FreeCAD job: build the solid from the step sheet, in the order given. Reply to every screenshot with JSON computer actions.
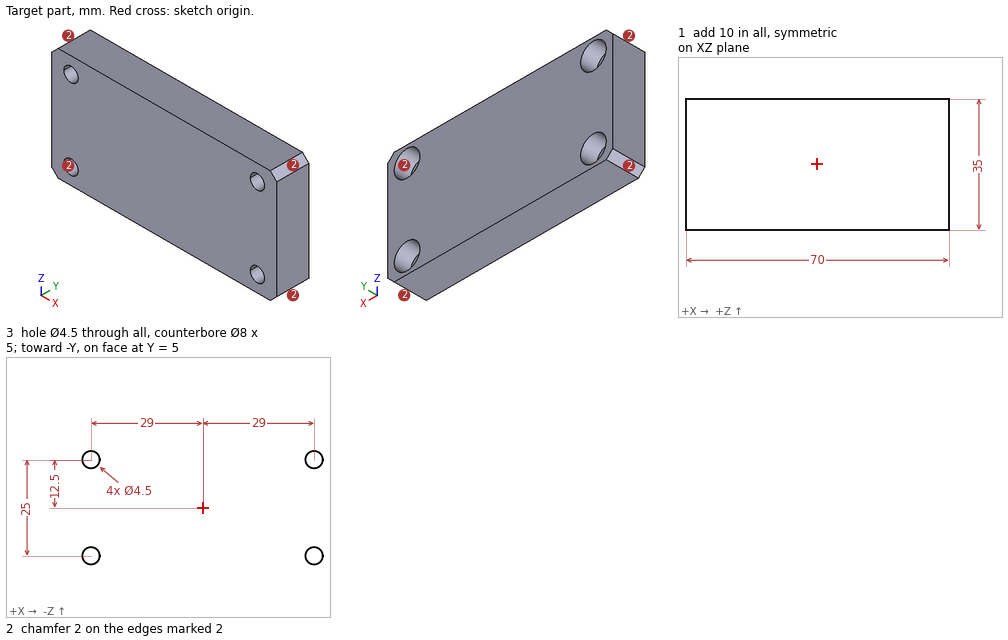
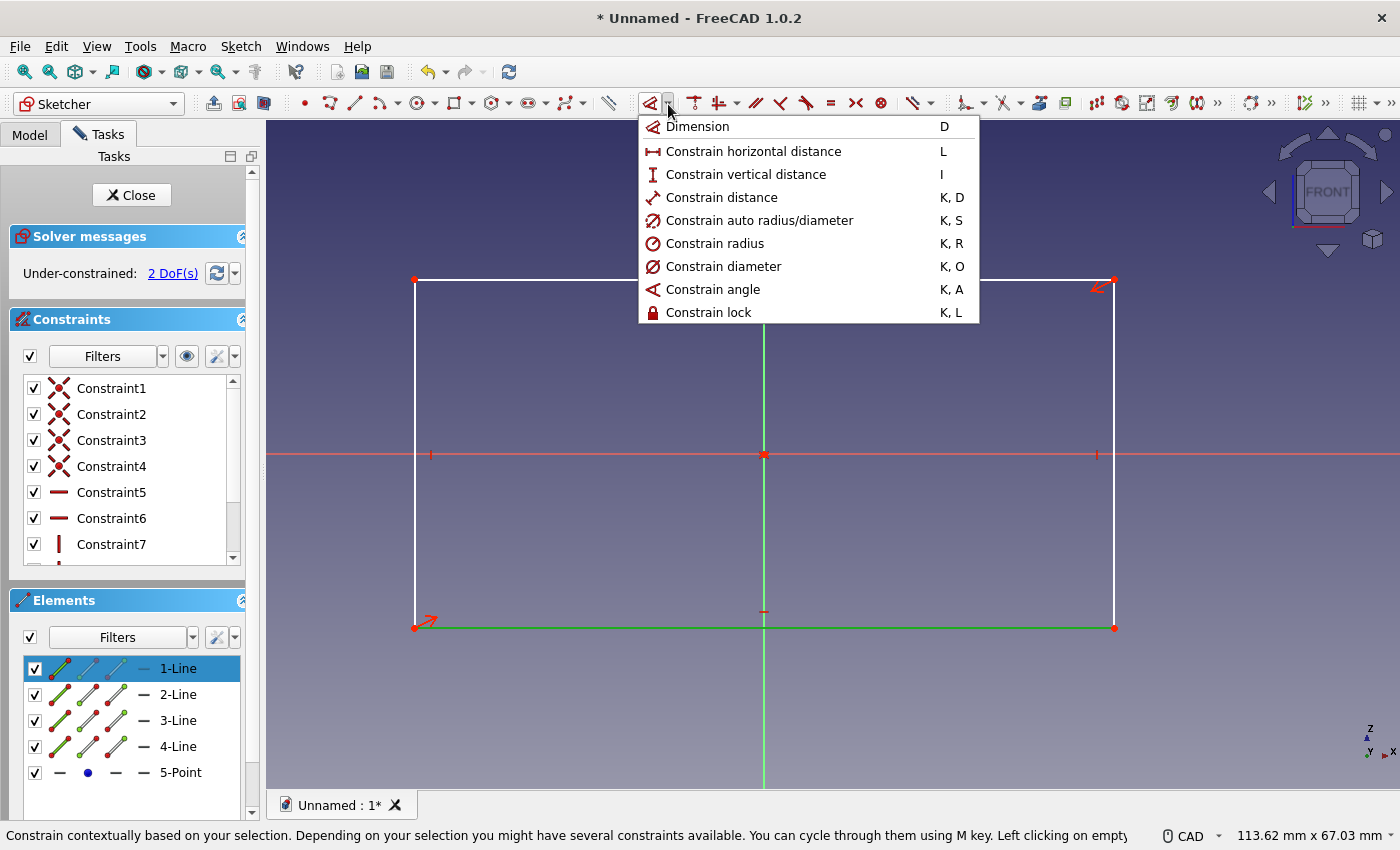
{"action": "left_click", "coordinate": [809, 152]}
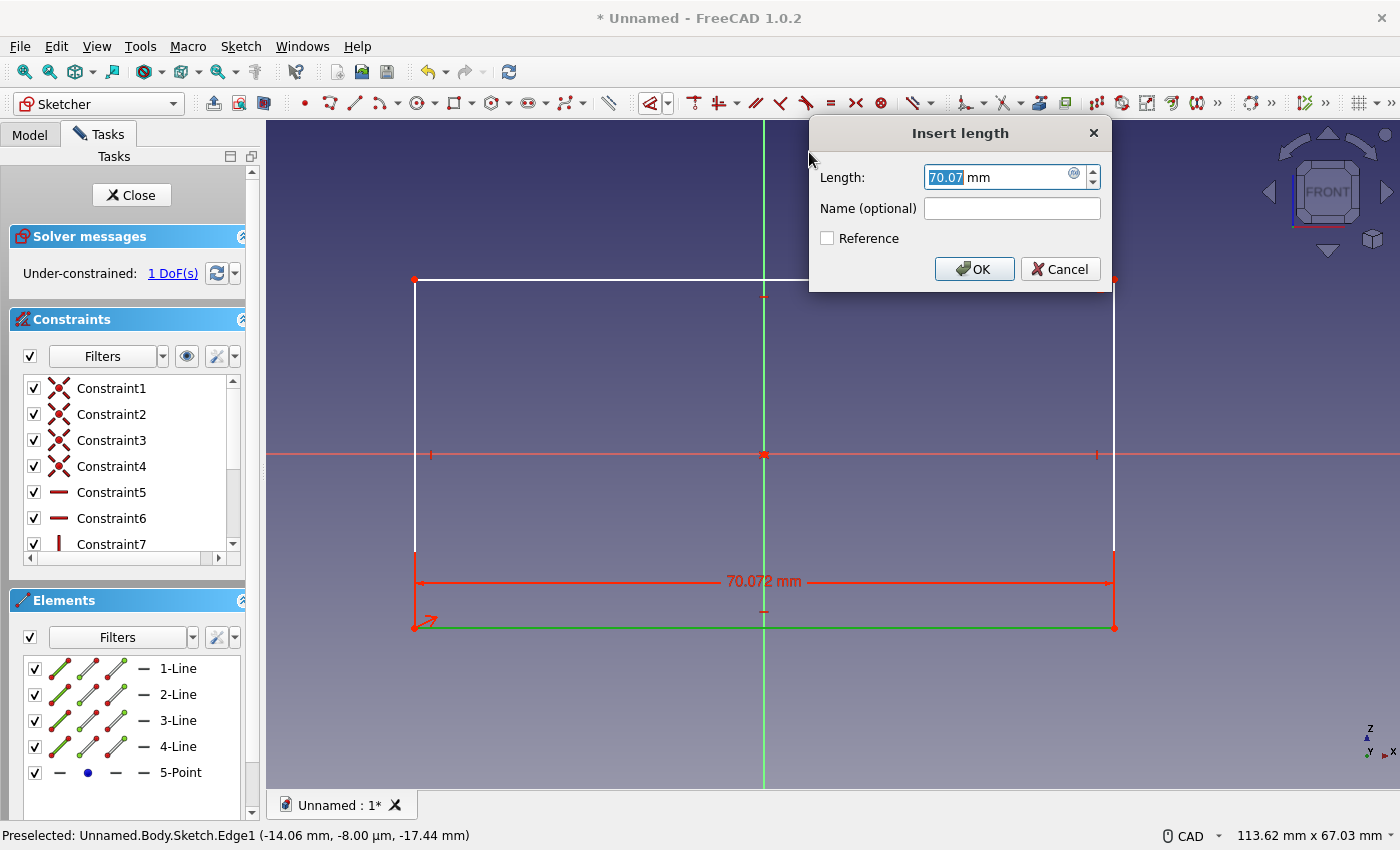
{"action": "type", "text": "70"}
{"action": "key", "text": "Return"}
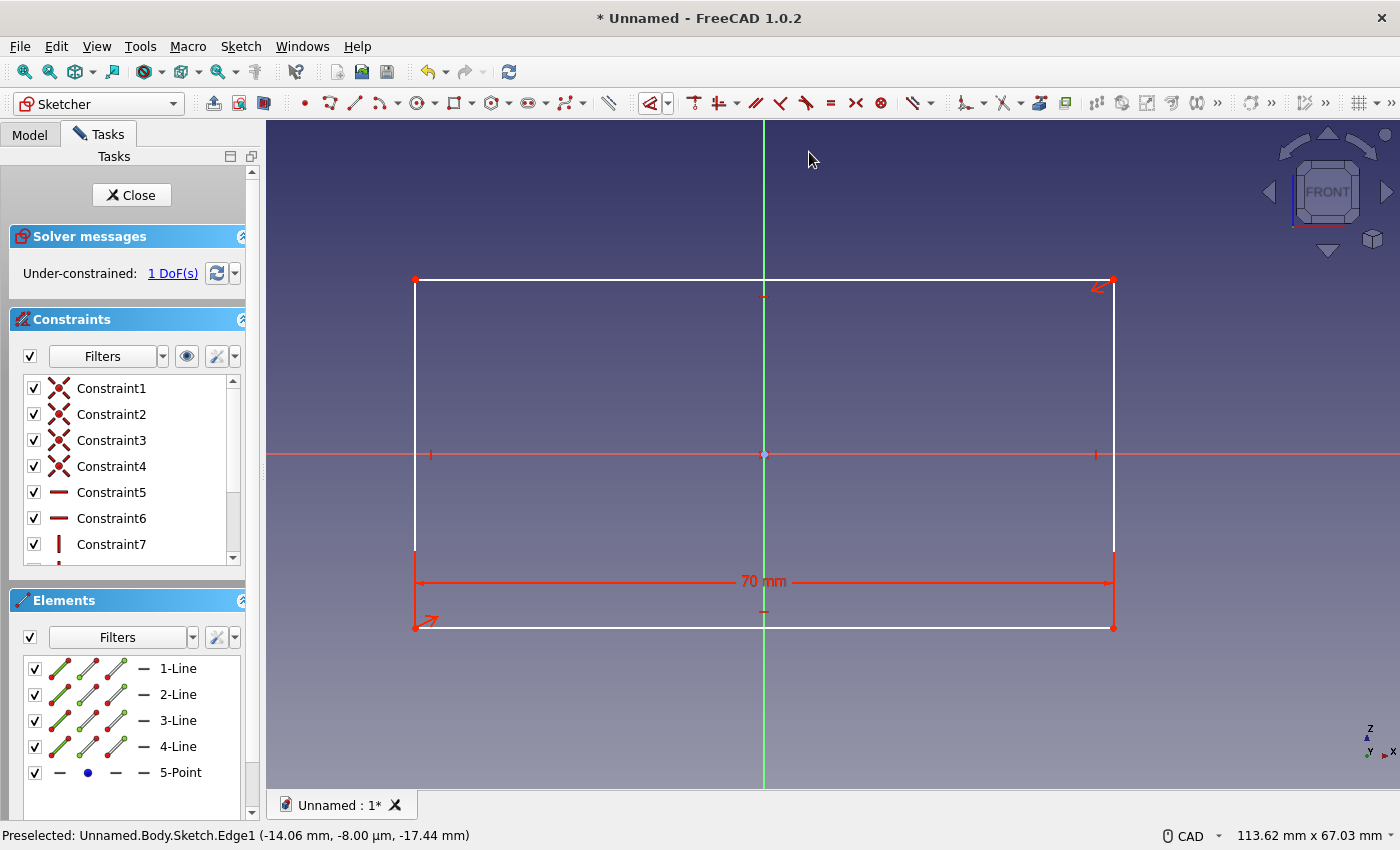
{"action": "left_click", "coordinate": [1114, 524]}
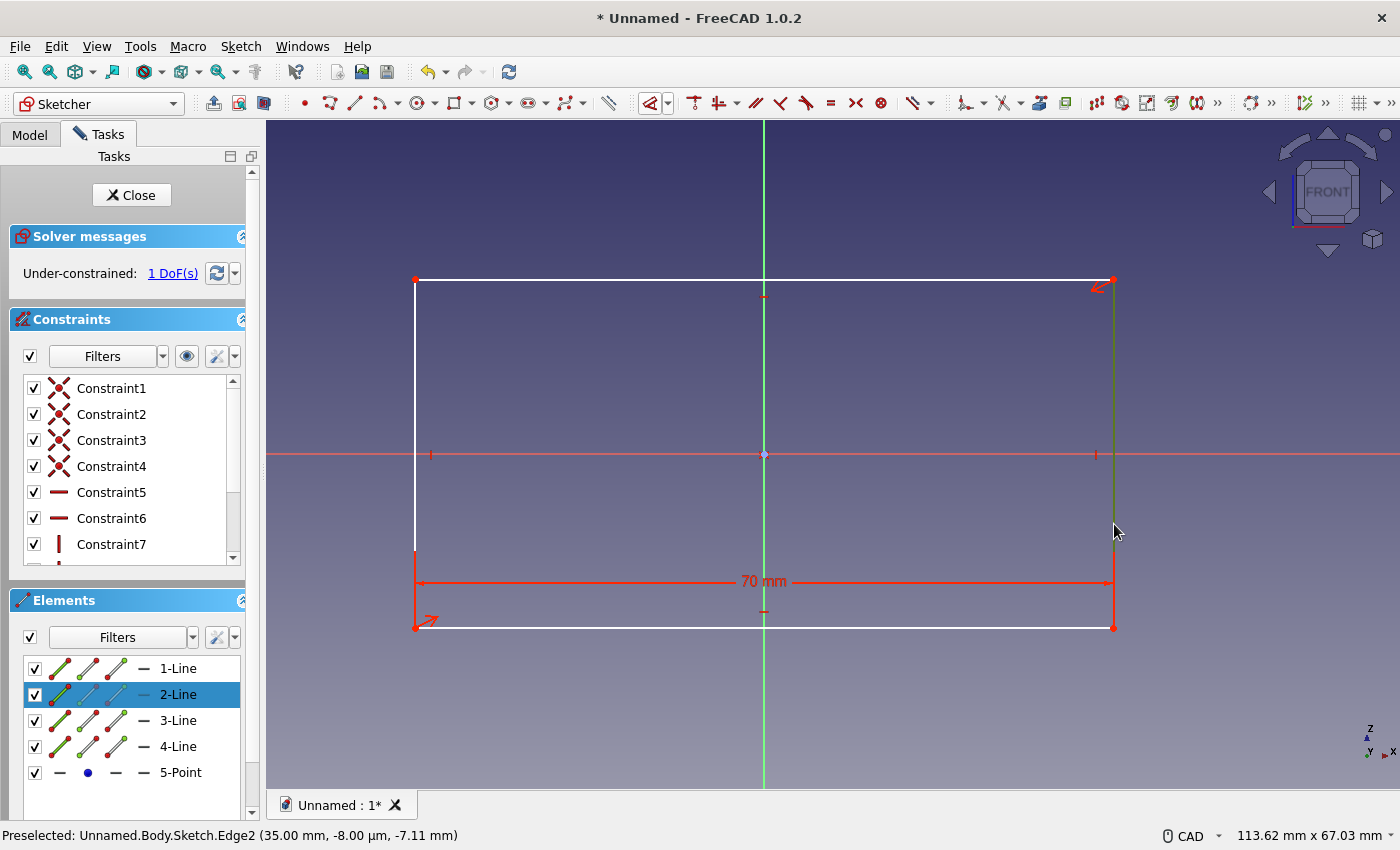
{"action": "left_click", "coordinate": [668, 104]}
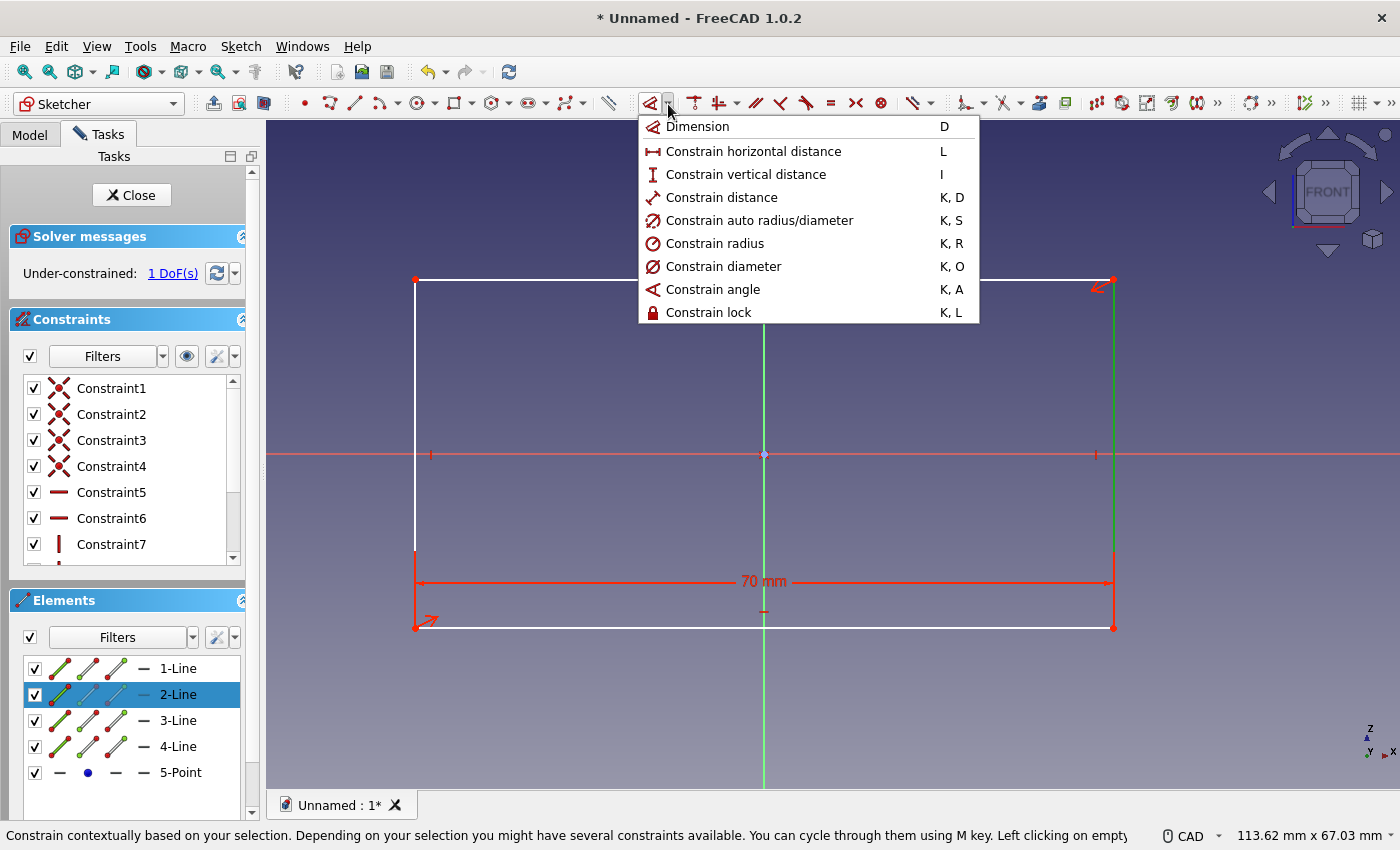
{"action": "left_click", "coordinate": [809, 174]}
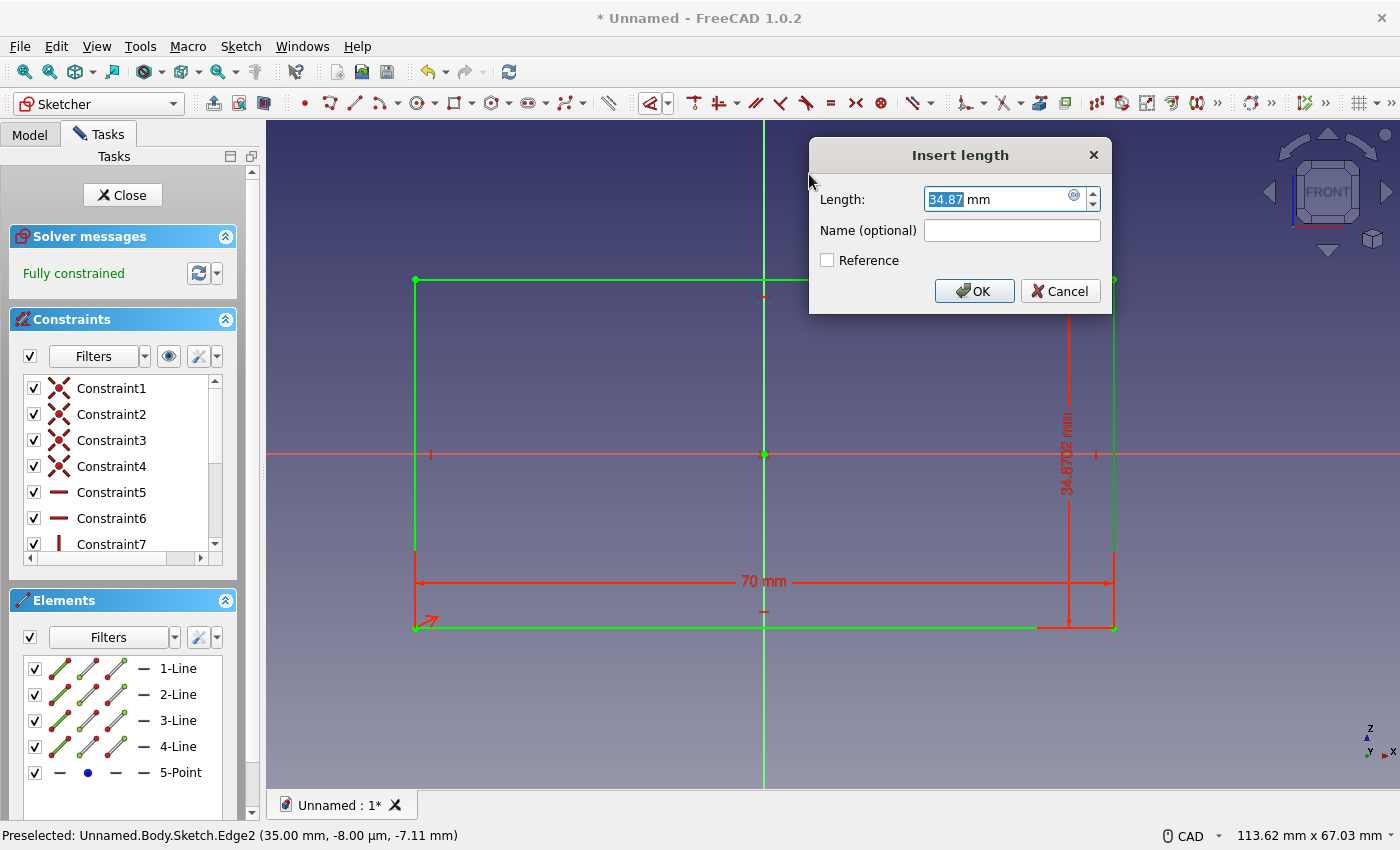
{"action": "type", "text": "35"}
{"action": "key", "text": "Return"}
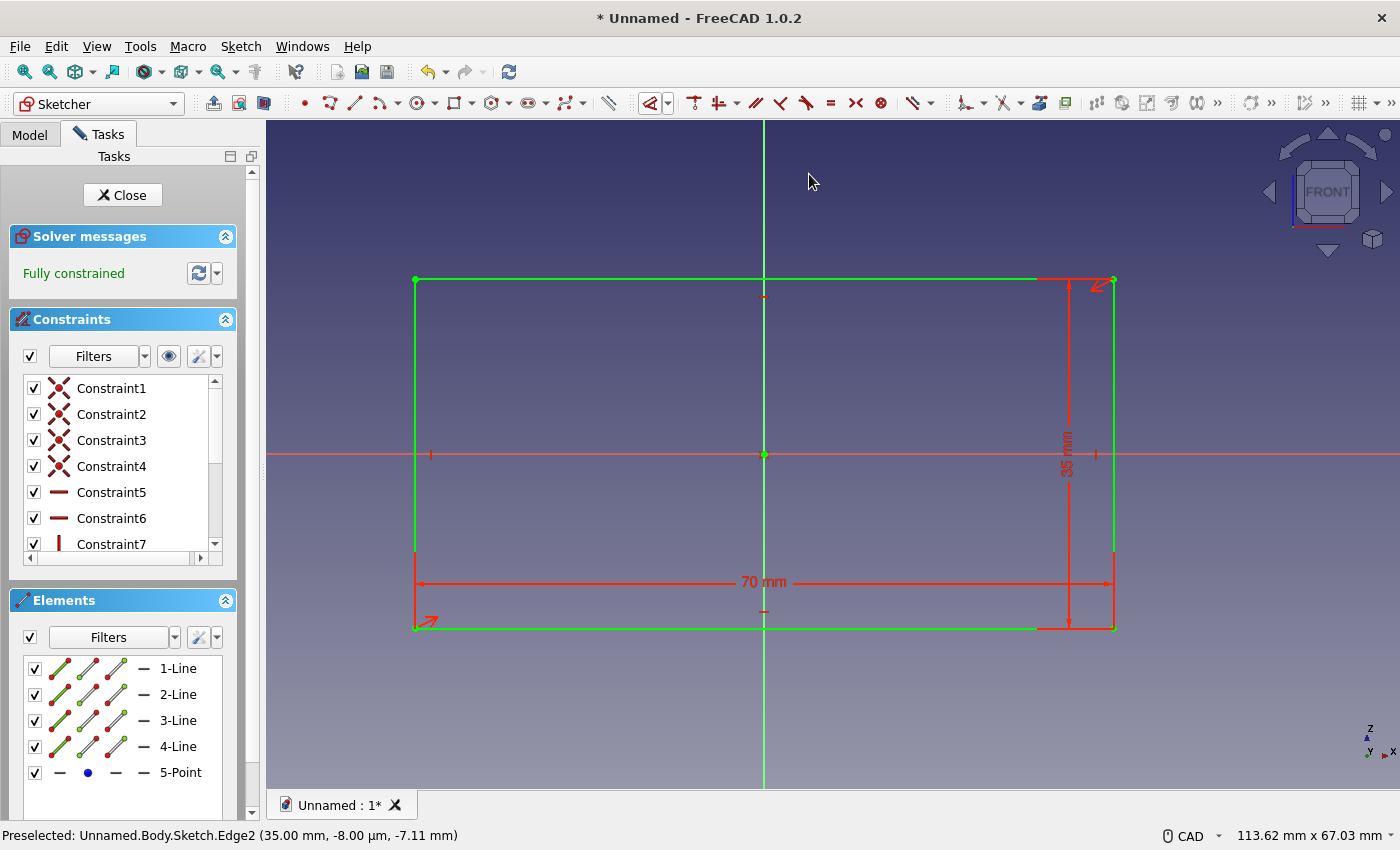
{"action": "left_click", "coordinate": [123, 195]}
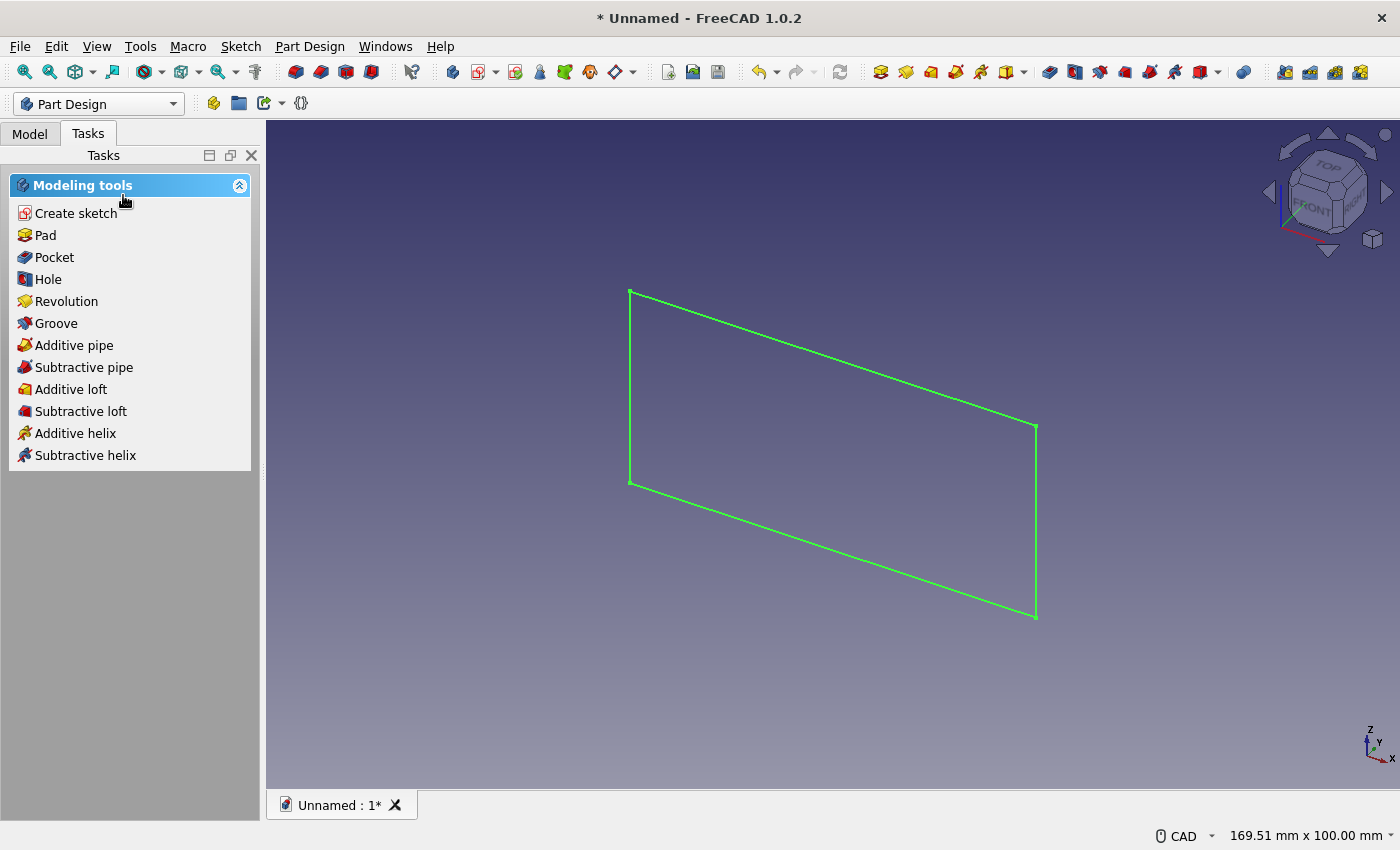
{"action": "left_click", "coordinate": [881, 72]}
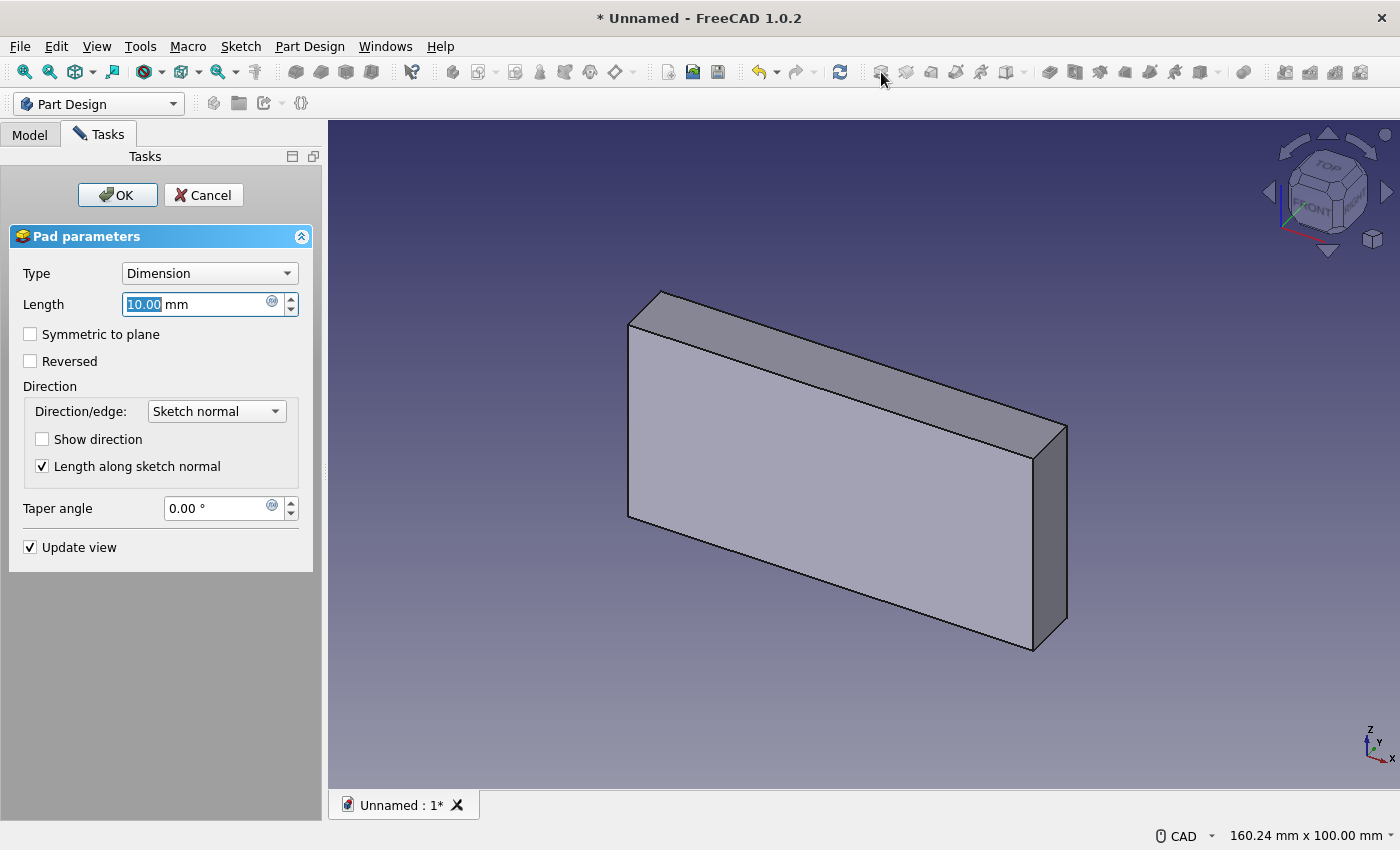
{"action": "type", "text": "10"}
{"action": "key", "text": "Tab"}